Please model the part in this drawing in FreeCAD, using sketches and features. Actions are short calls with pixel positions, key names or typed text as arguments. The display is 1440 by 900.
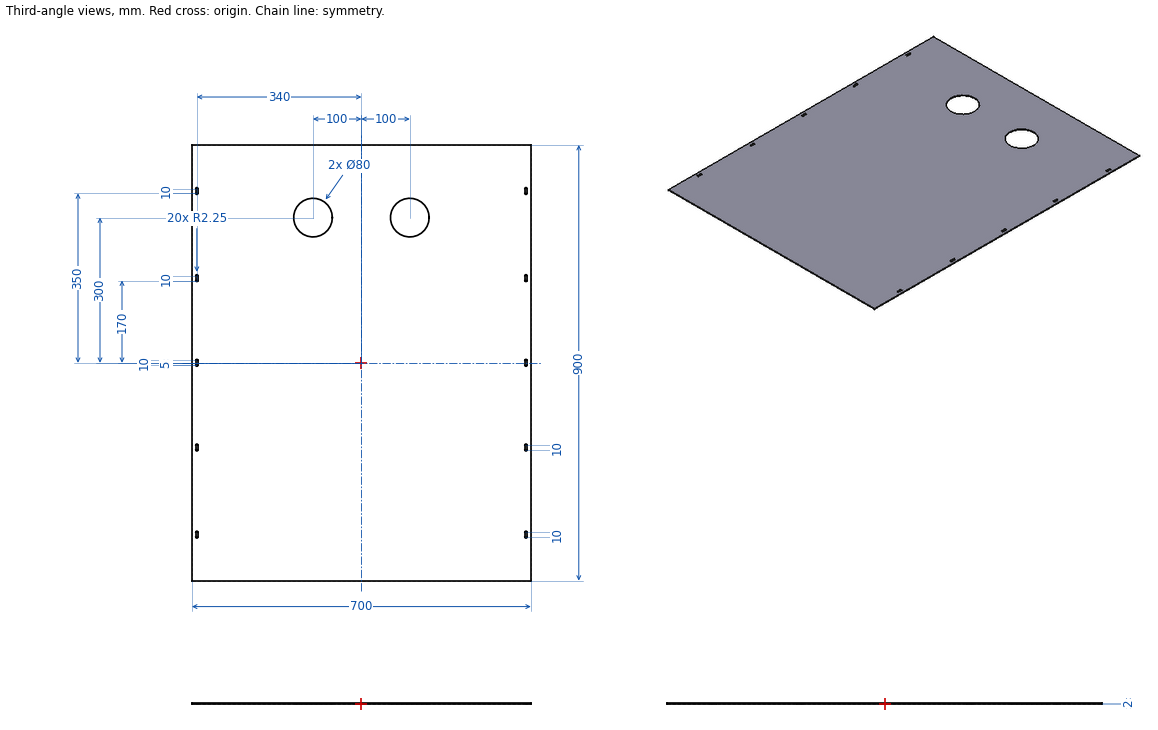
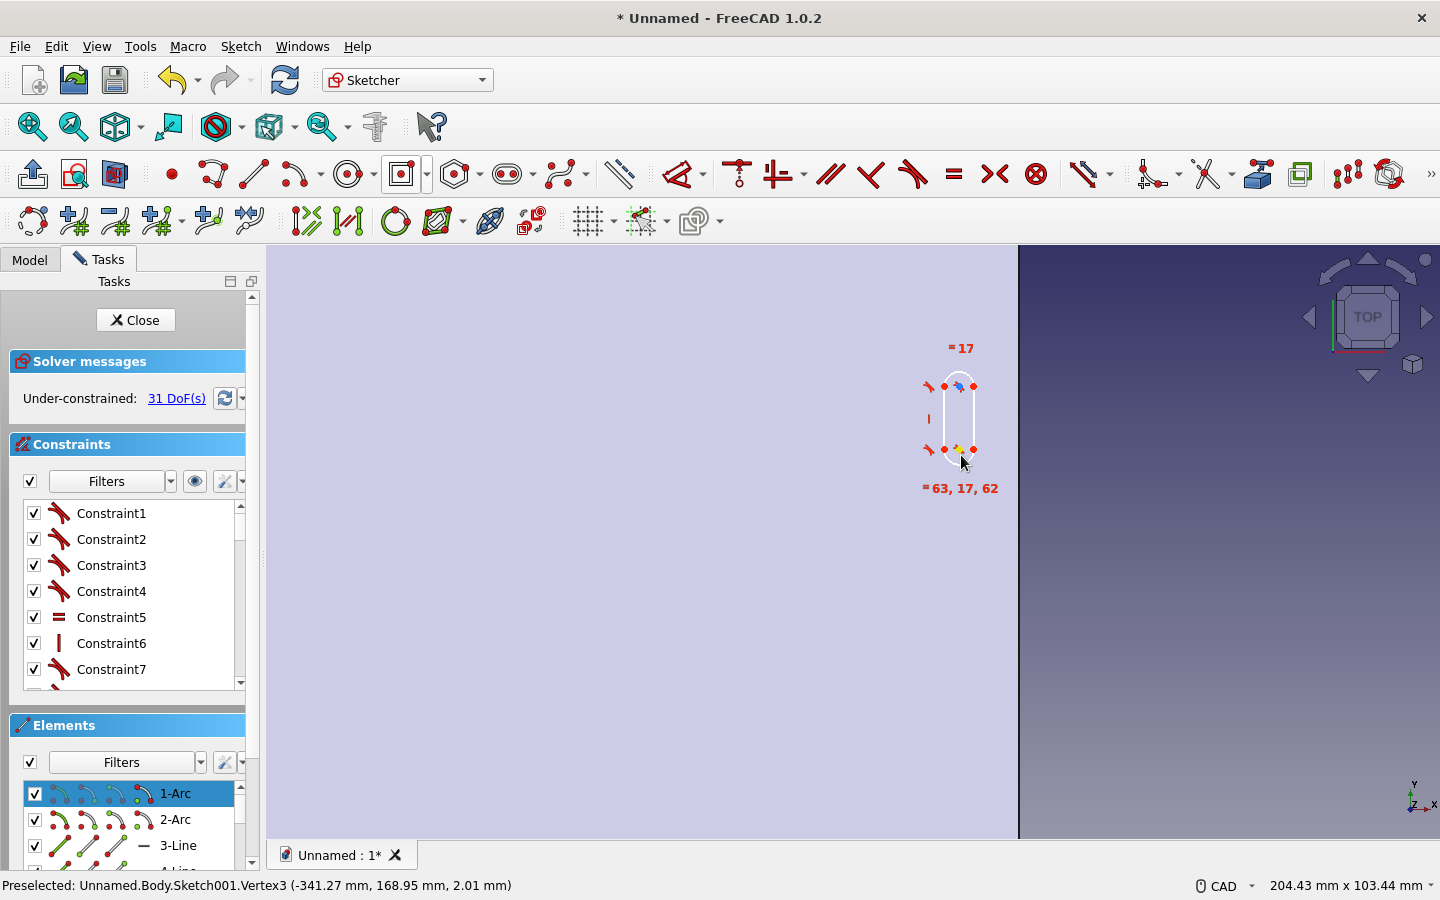
click(959, 450)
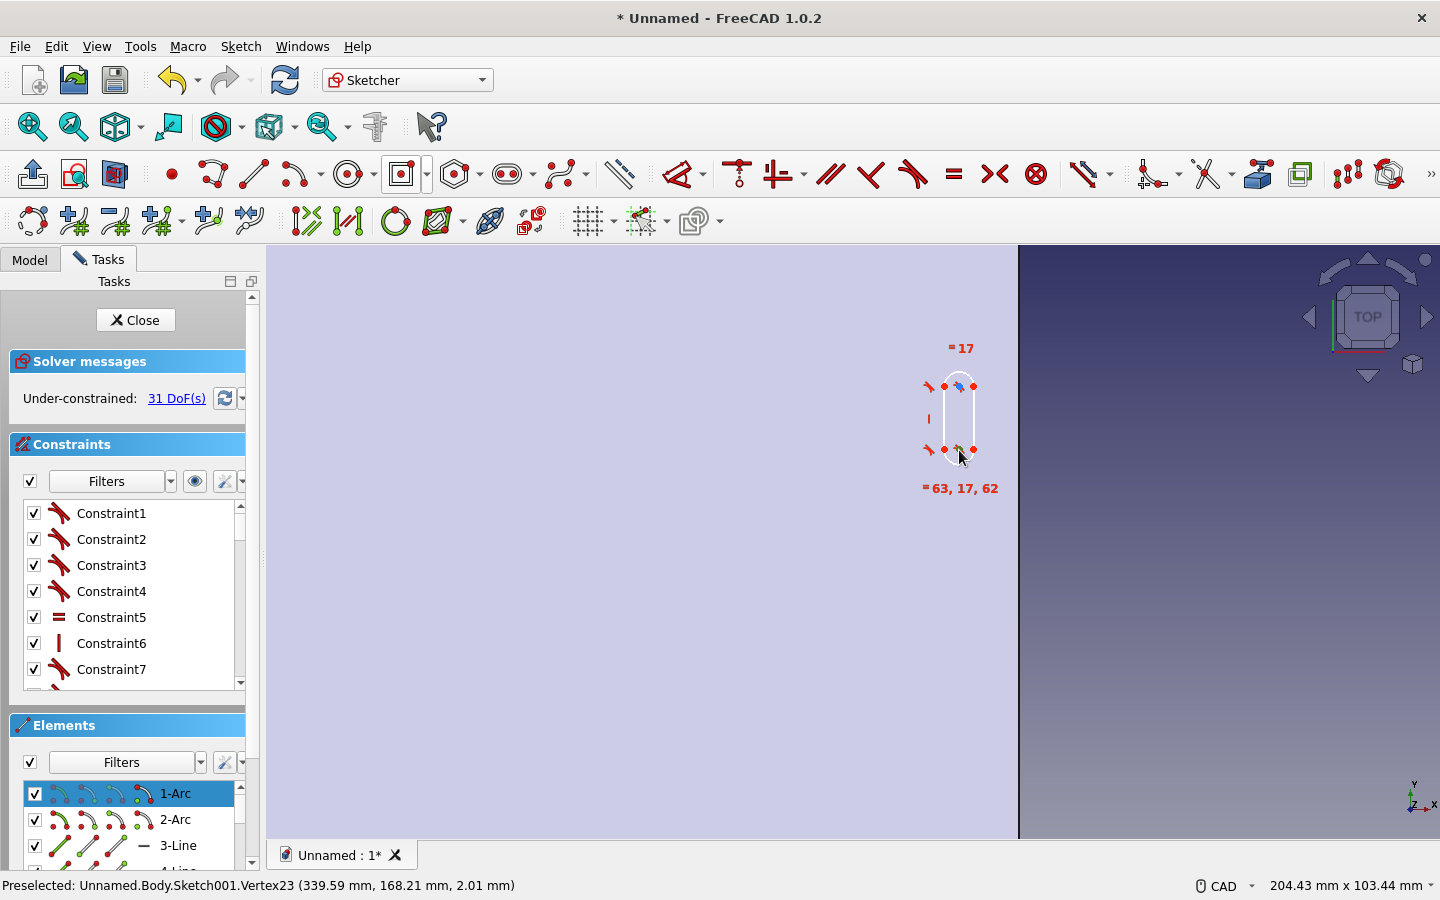
scroll(962, 455, down, 12)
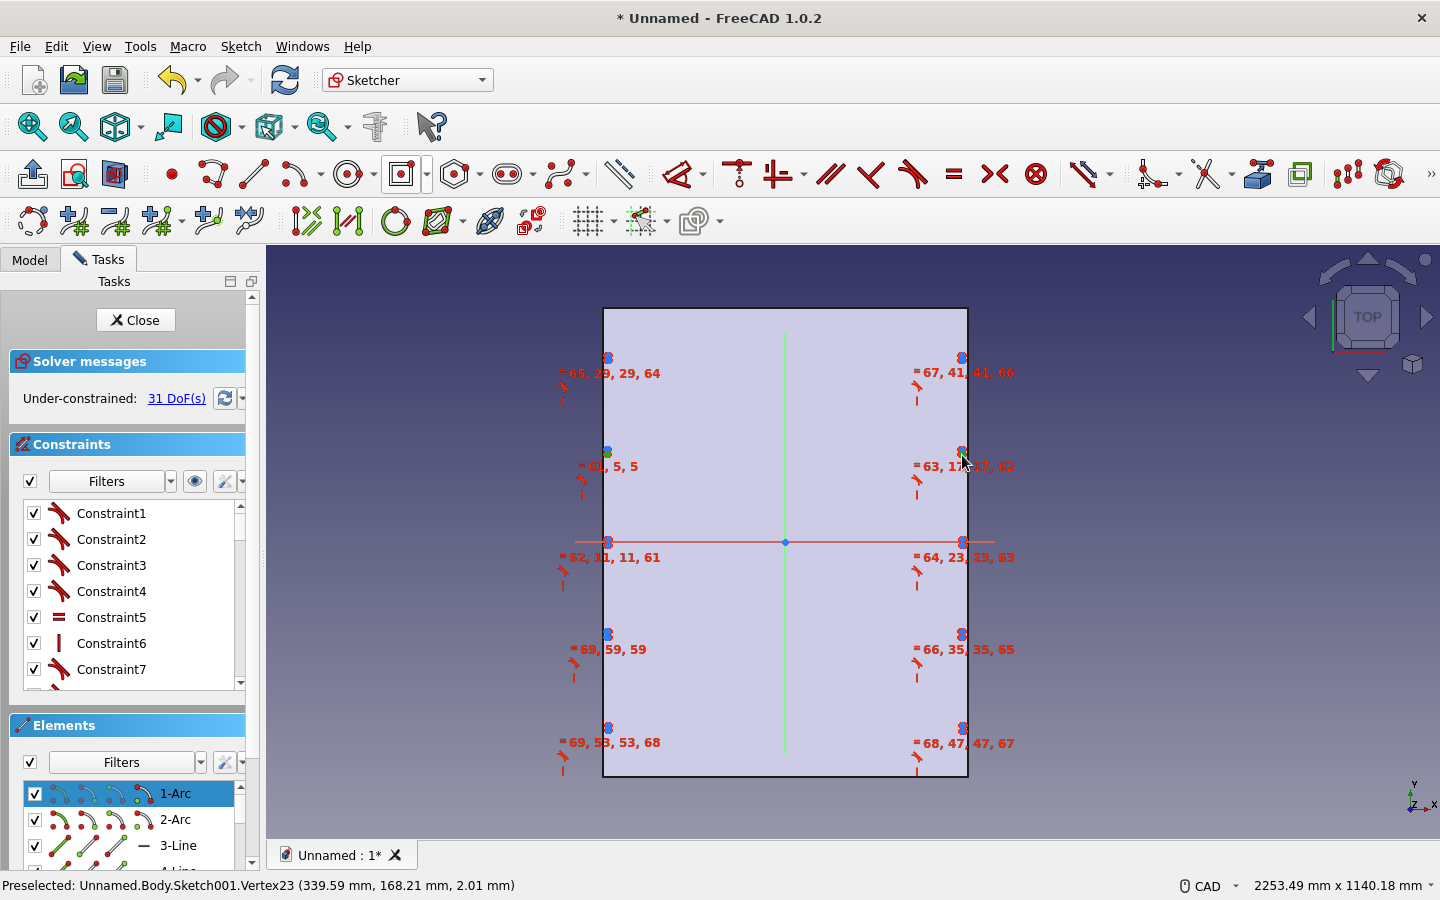
click(785, 734)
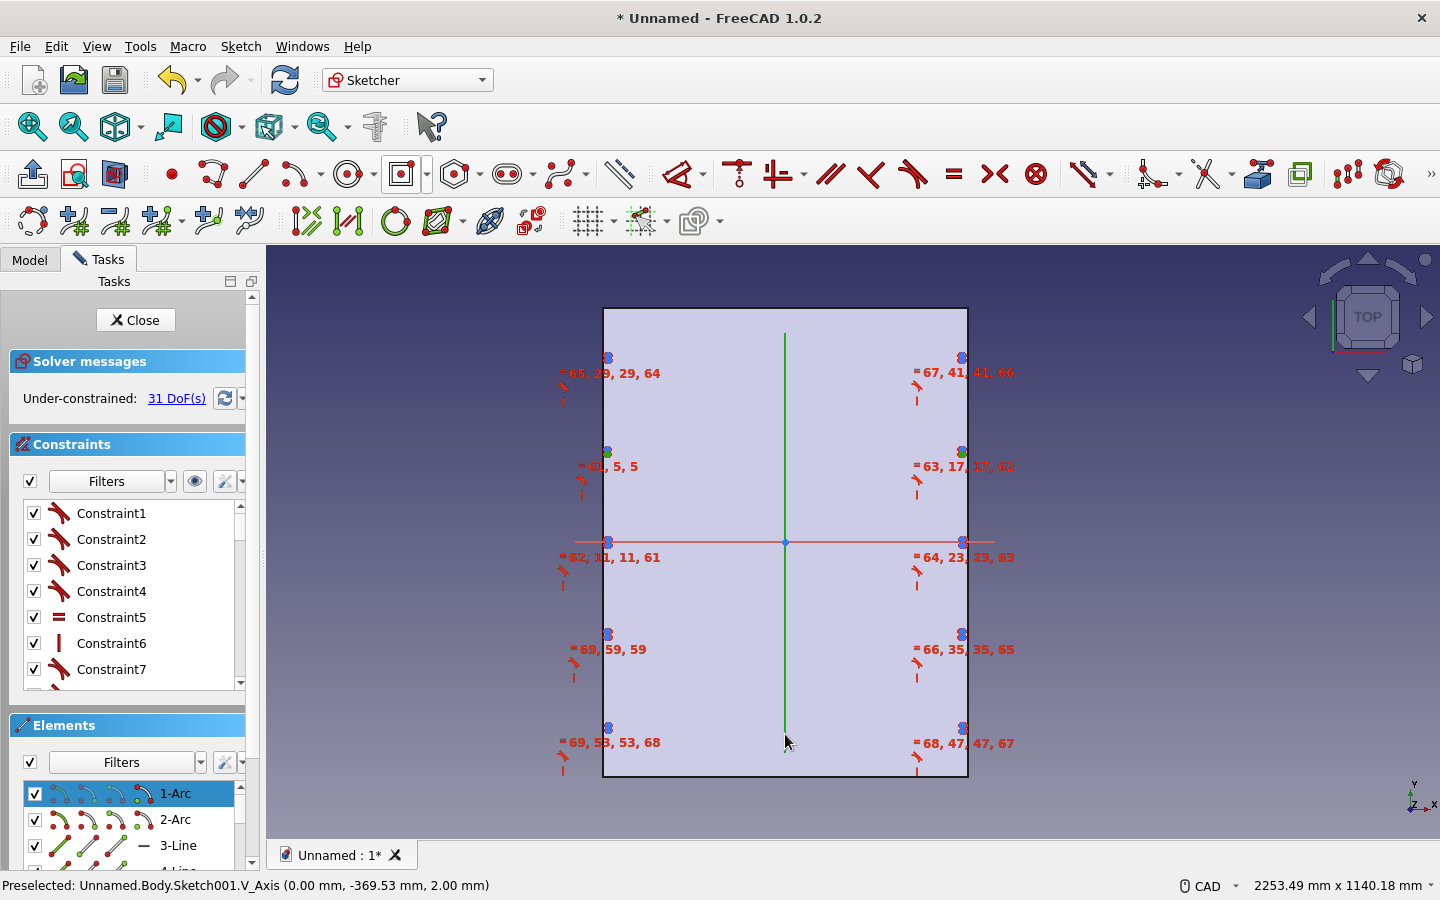
click(995, 174)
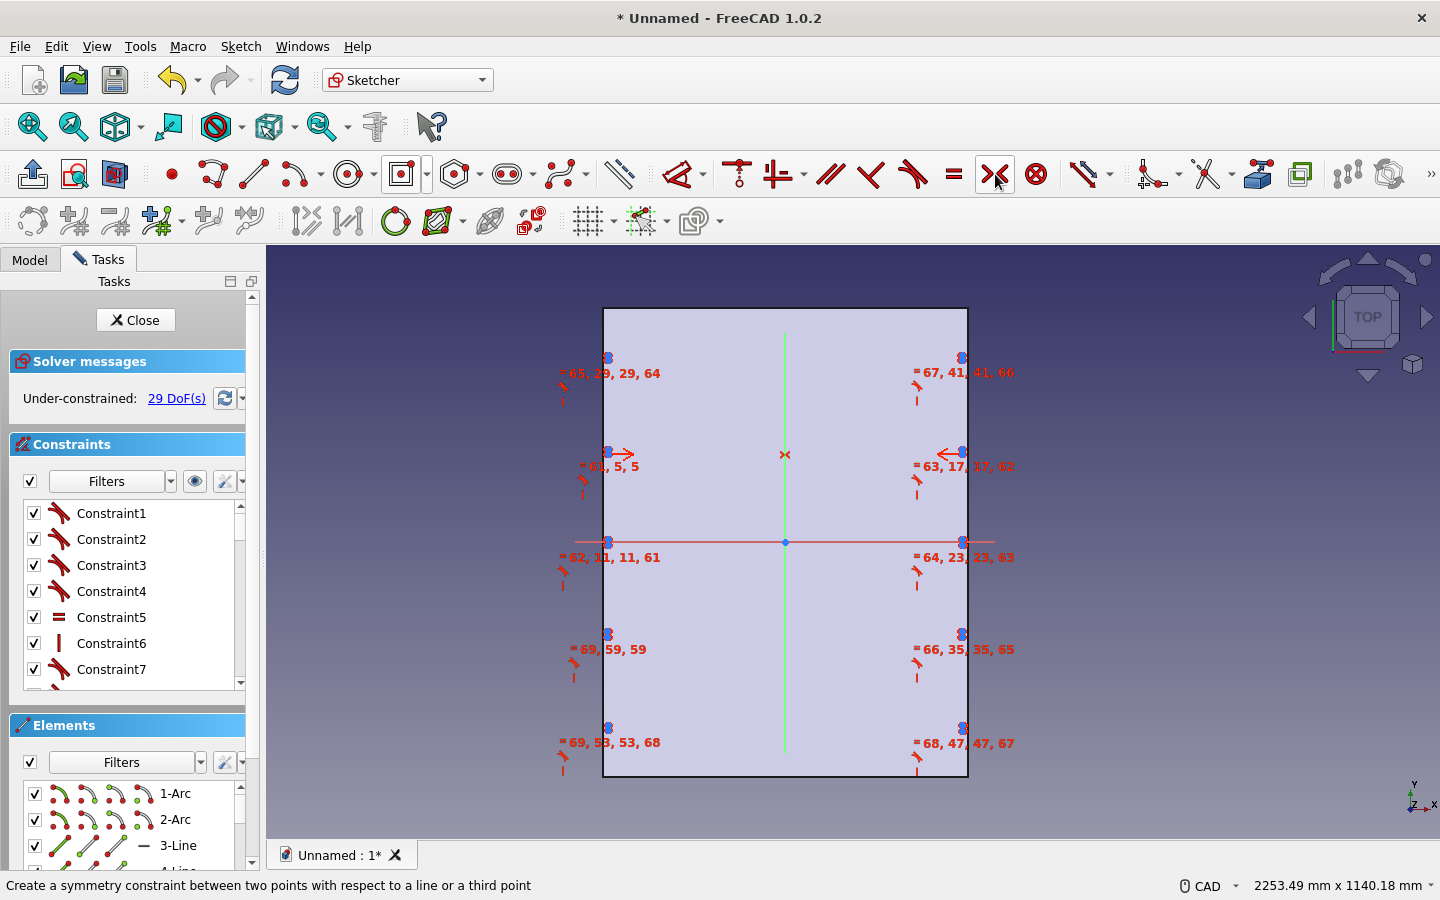
scroll(608, 545, up, 12)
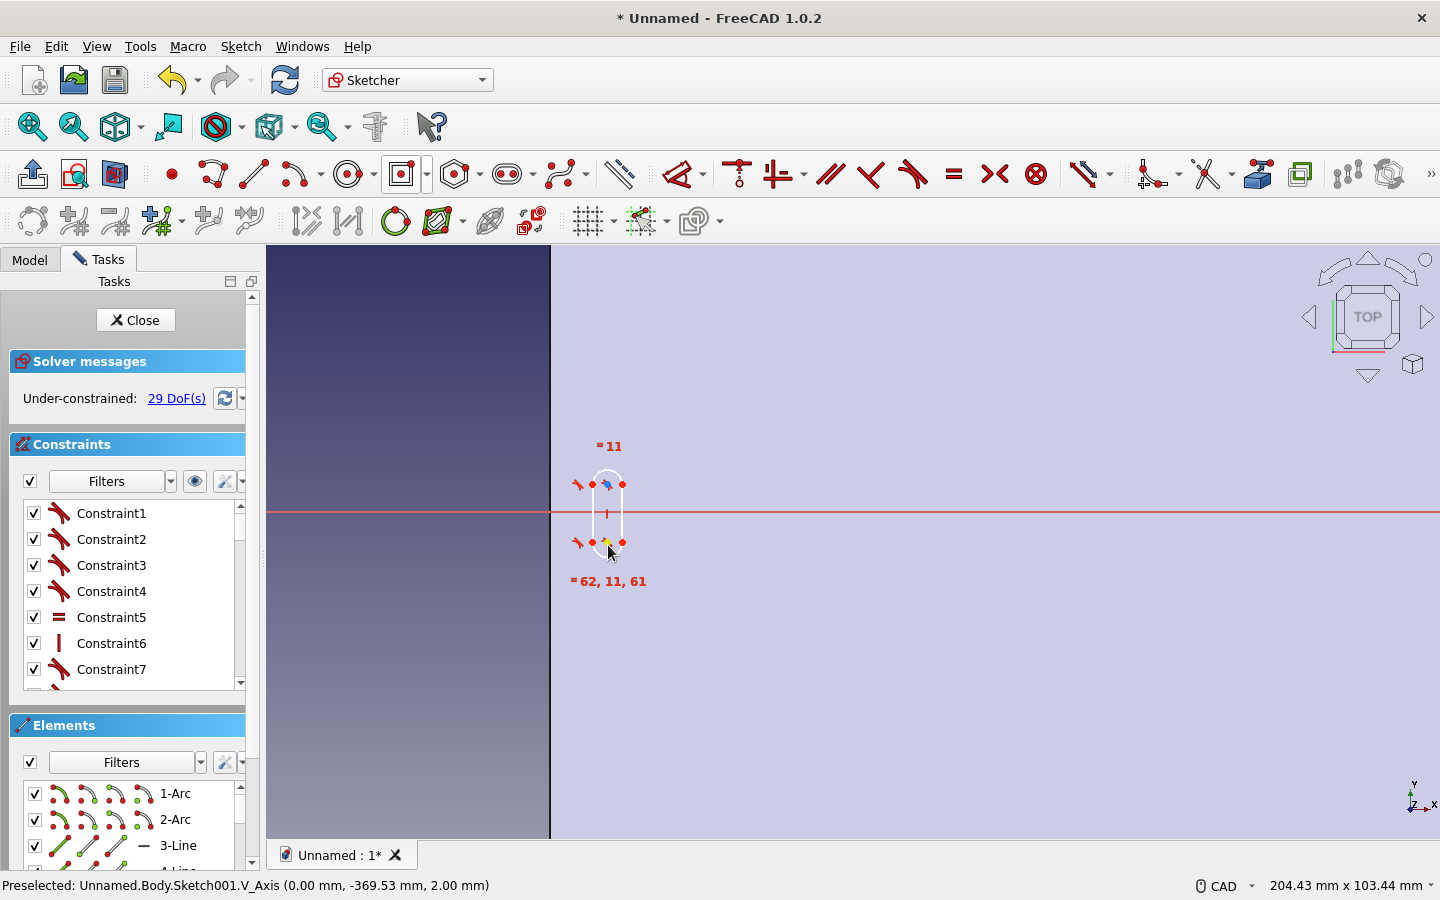
click(608, 543)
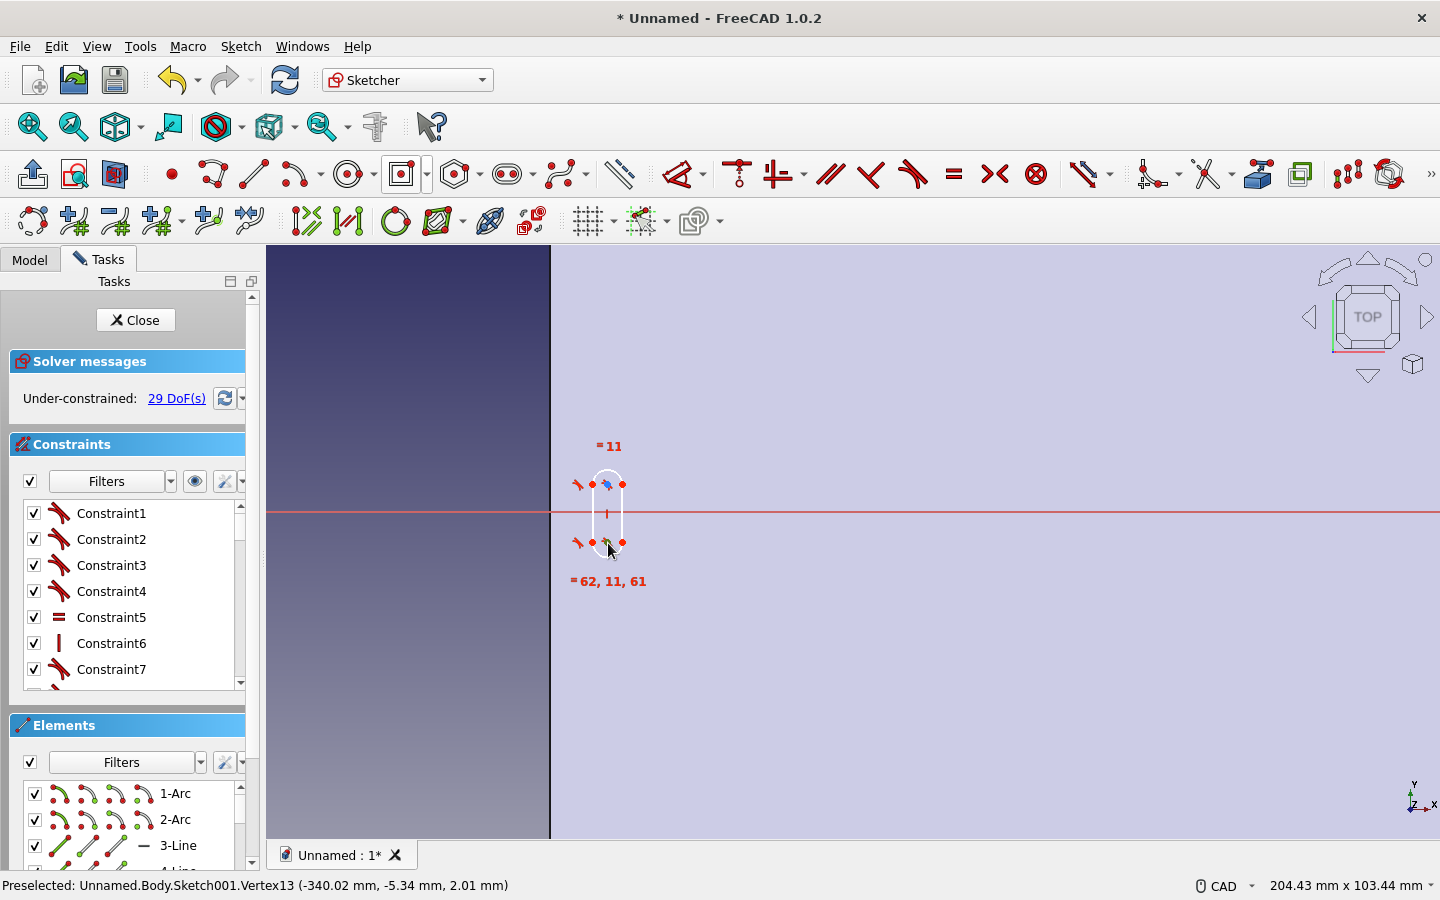
scroll(607, 545, down, 12)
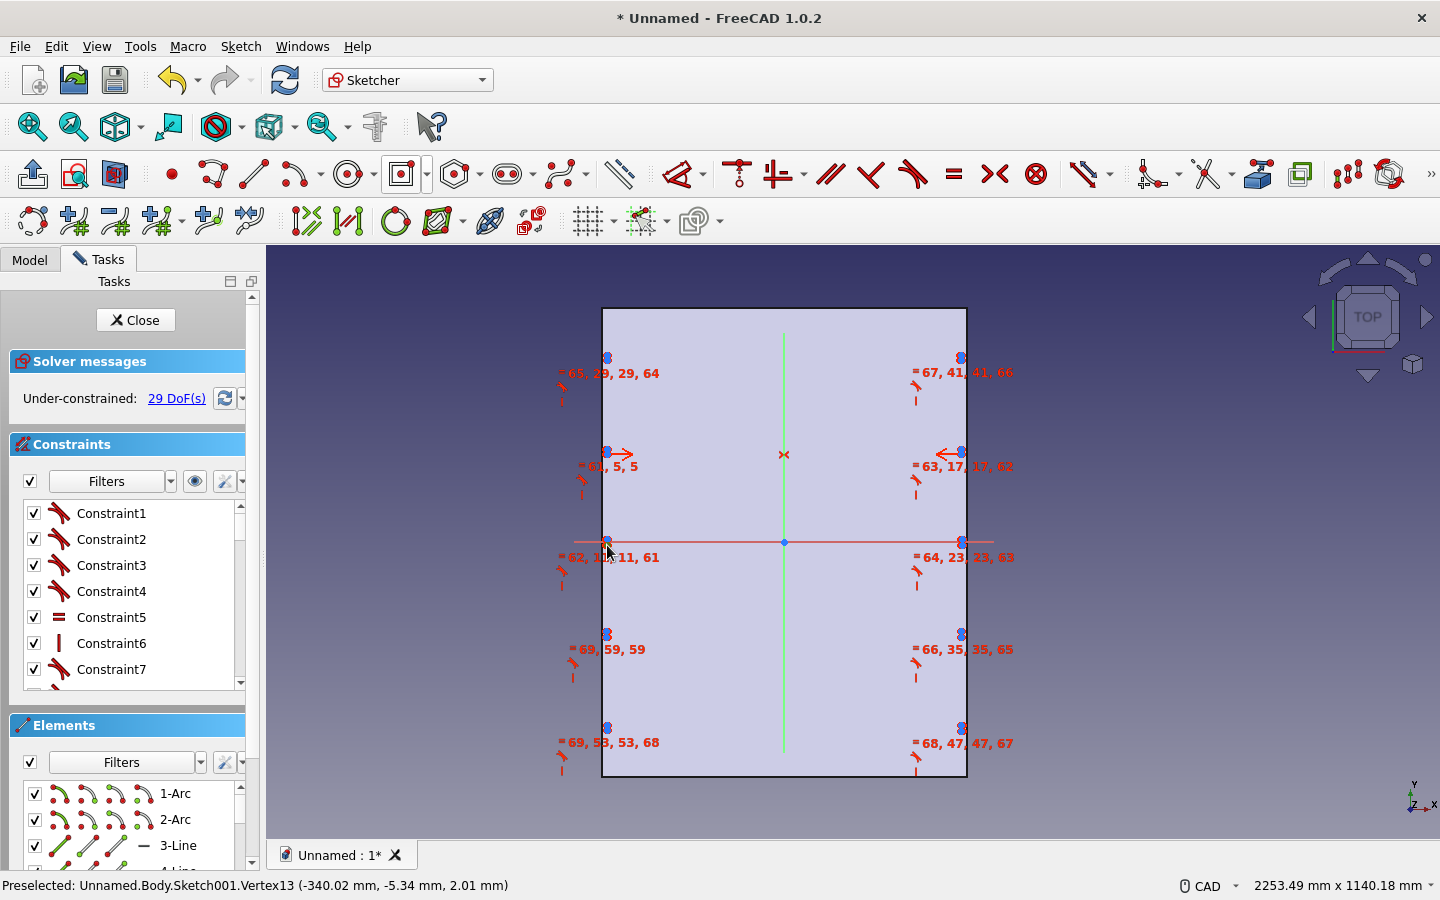
scroll(962, 545, up, 12)